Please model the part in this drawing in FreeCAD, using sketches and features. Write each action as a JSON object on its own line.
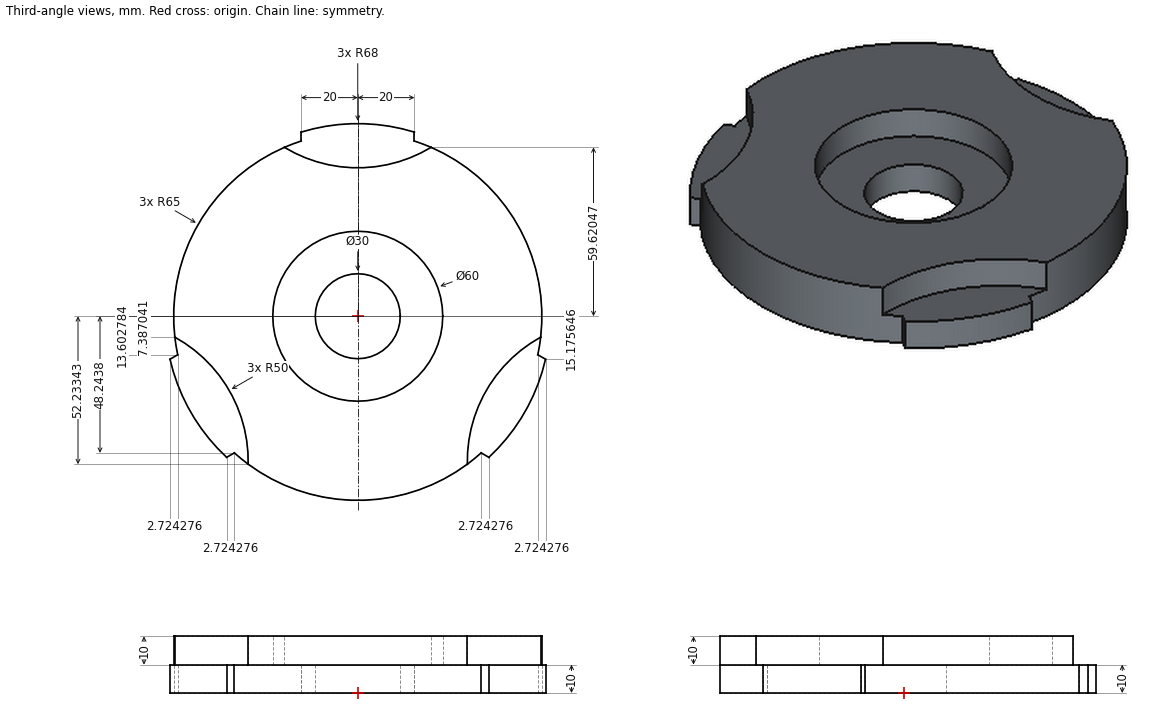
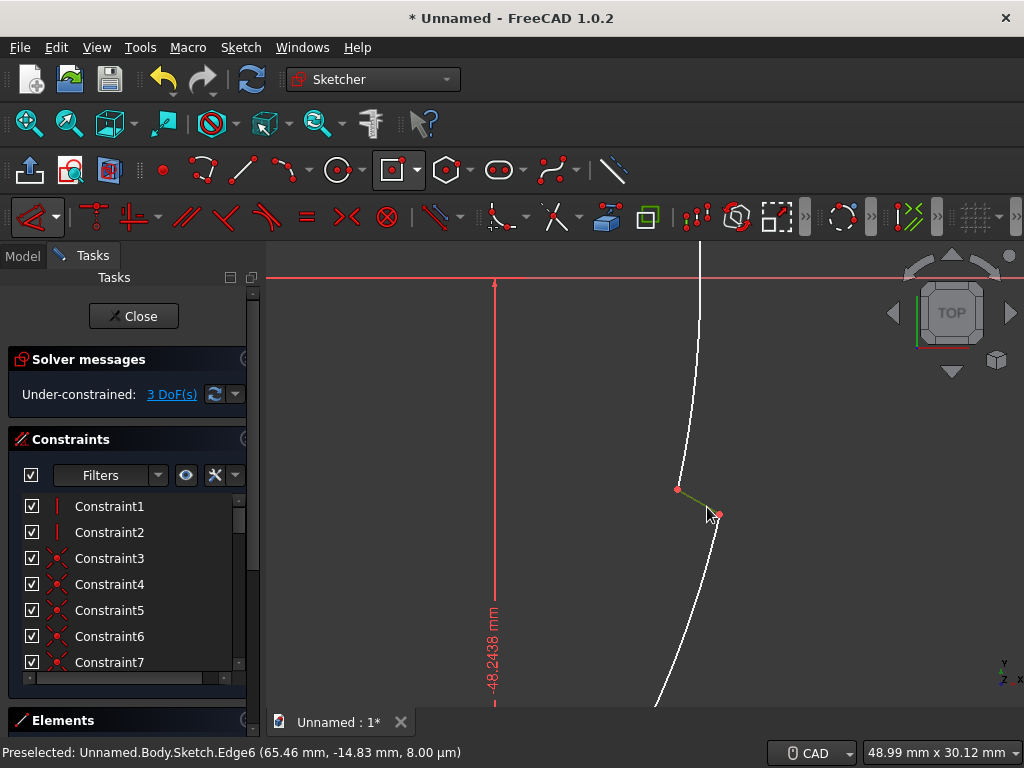
{"action": "key", "text": "l"}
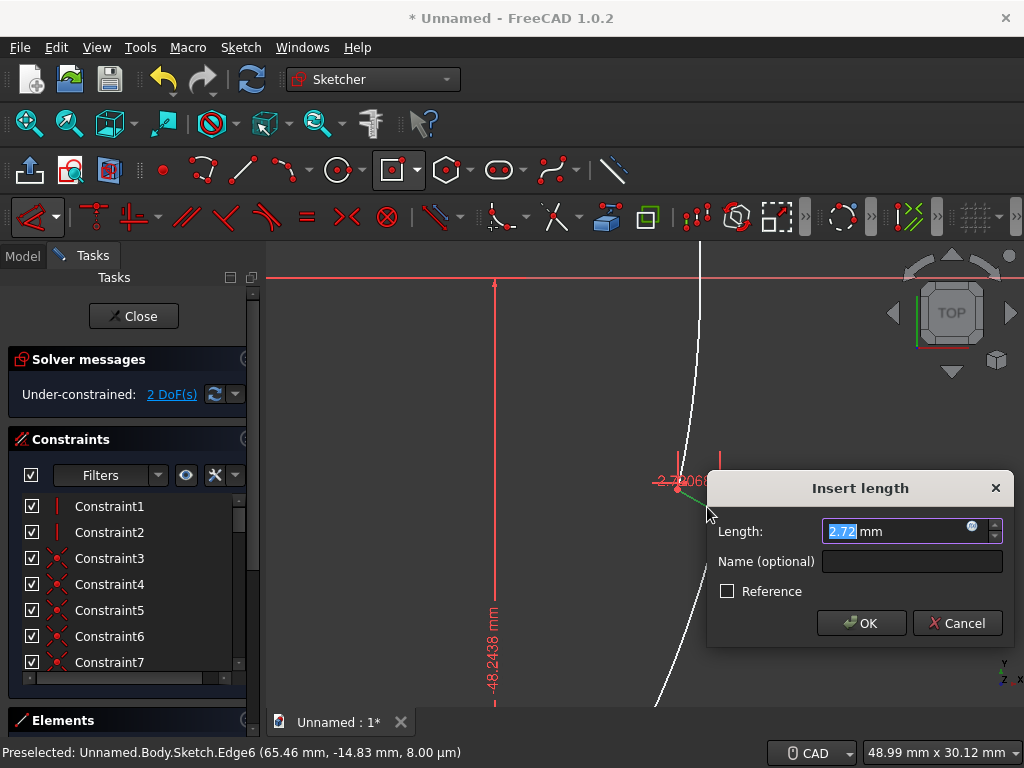
{"action": "type", "text": "2.724276"}
{"action": "key", "text": "Return"}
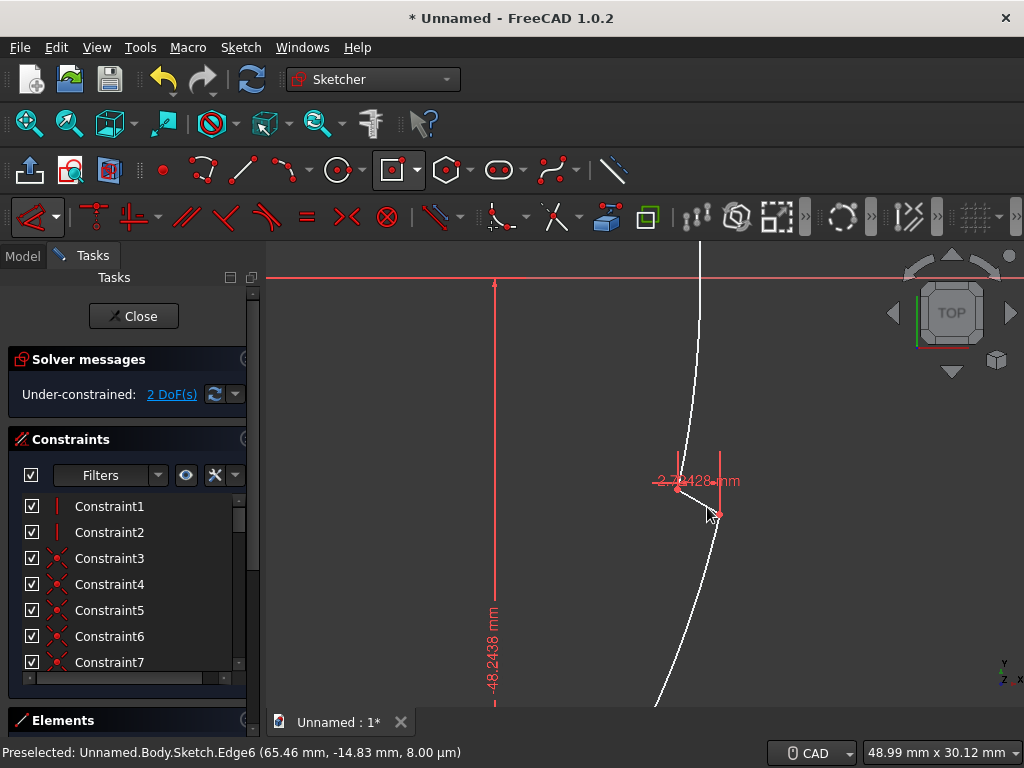
{"action": "scroll", "coordinate": [715, 508], "scroll_direction": "down", "scroll_amount": 10}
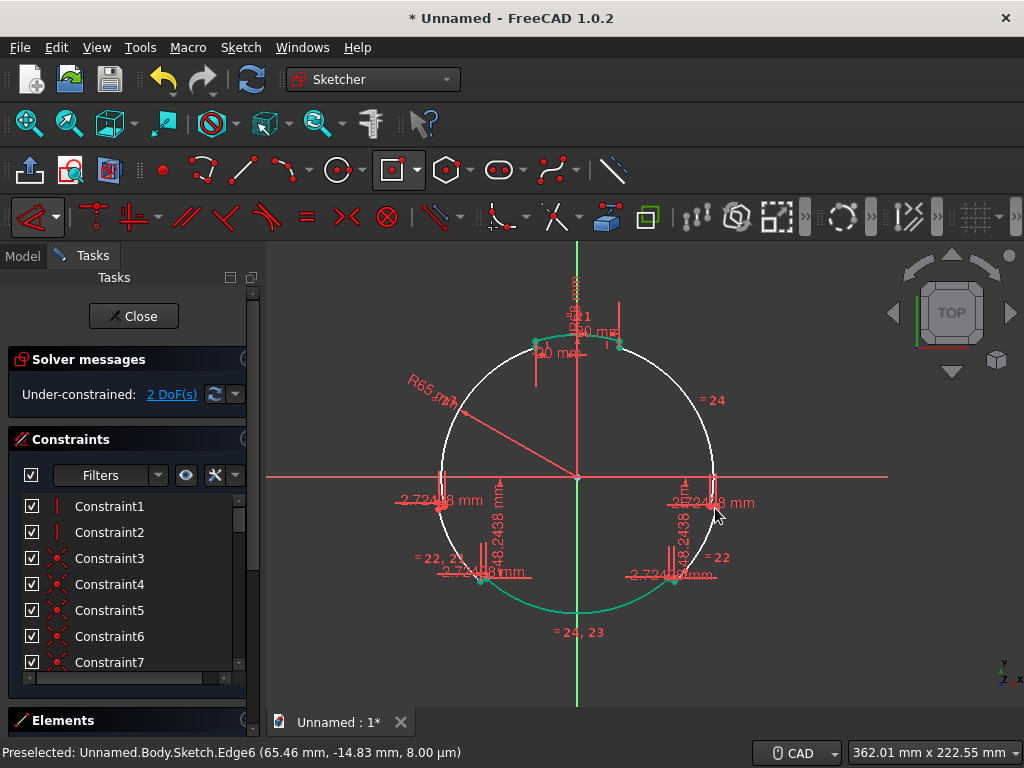
{"action": "scroll", "coordinate": [445, 507], "scroll_direction": "up", "scroll_amount": 4}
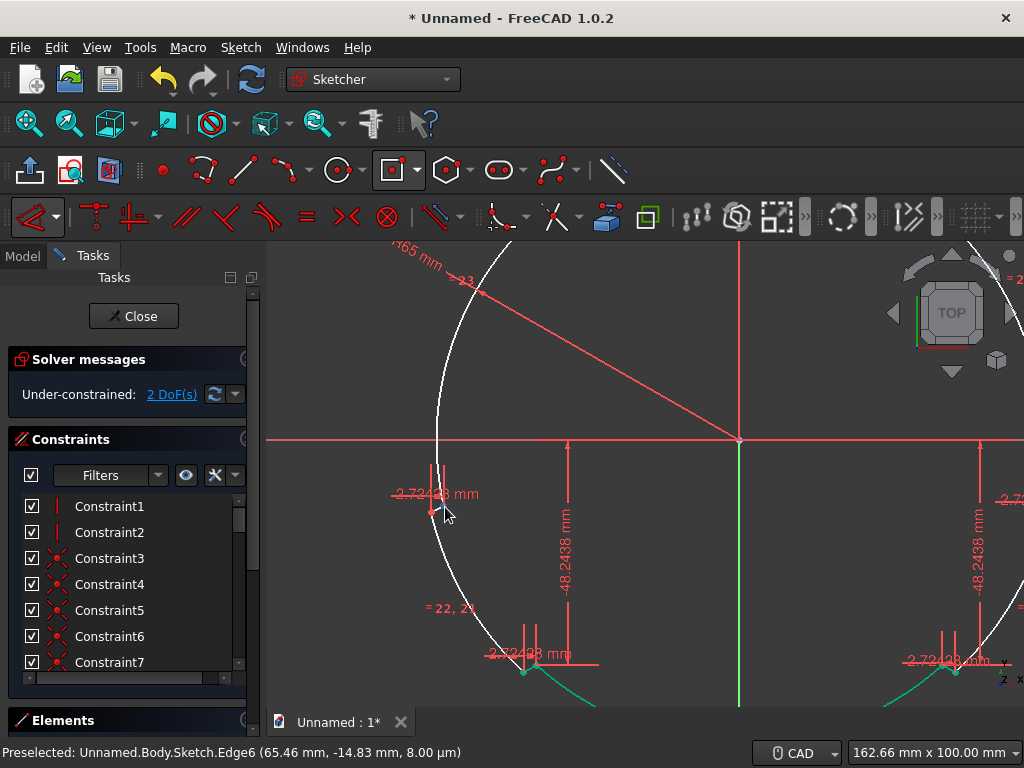
{"action": "left_click", "coordinate": [444, 506]}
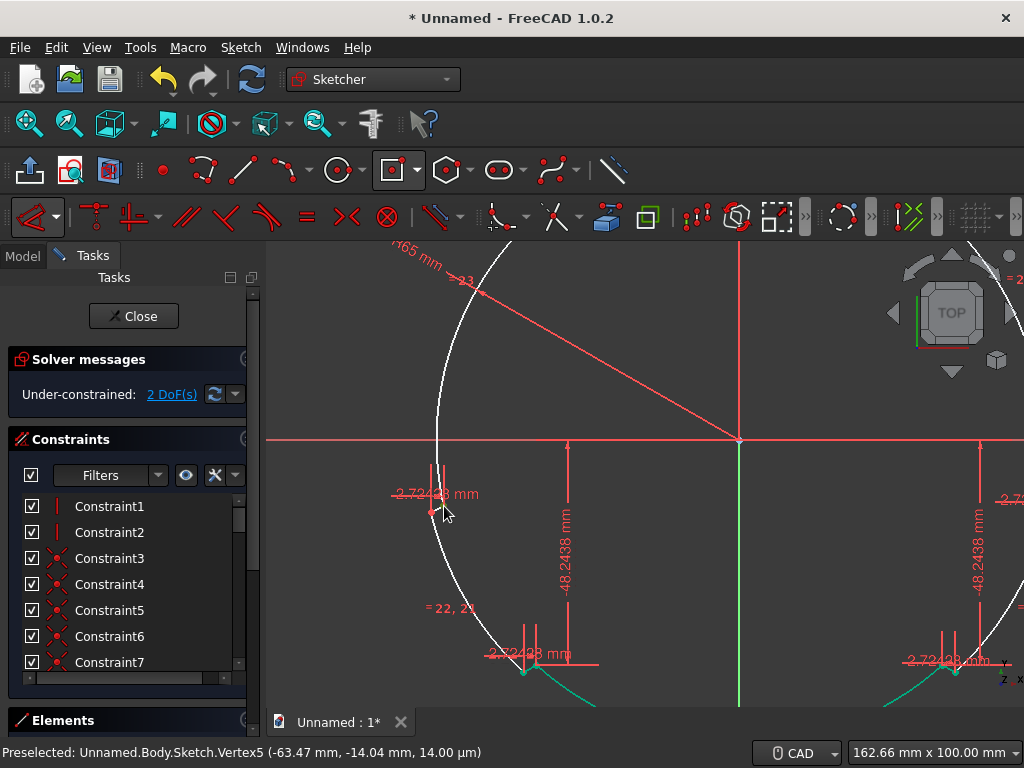
{"action": "key", "text": "i"}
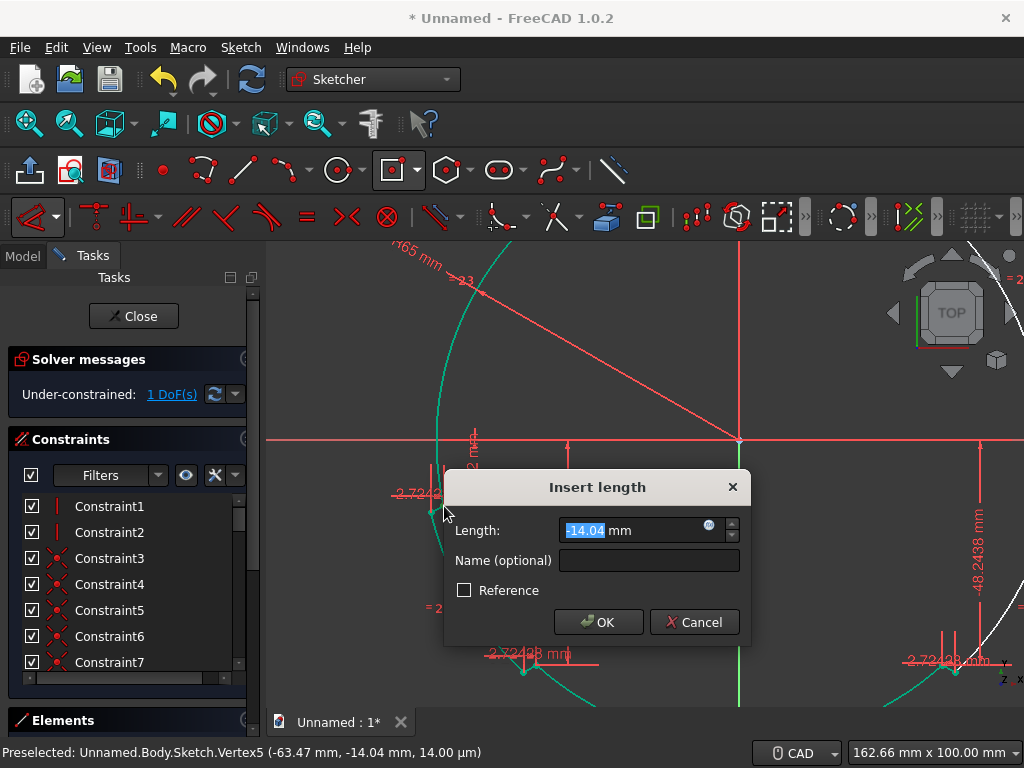
{"action": "type", "text": "-13.602784"}
{"action": "key", "text": "Return"}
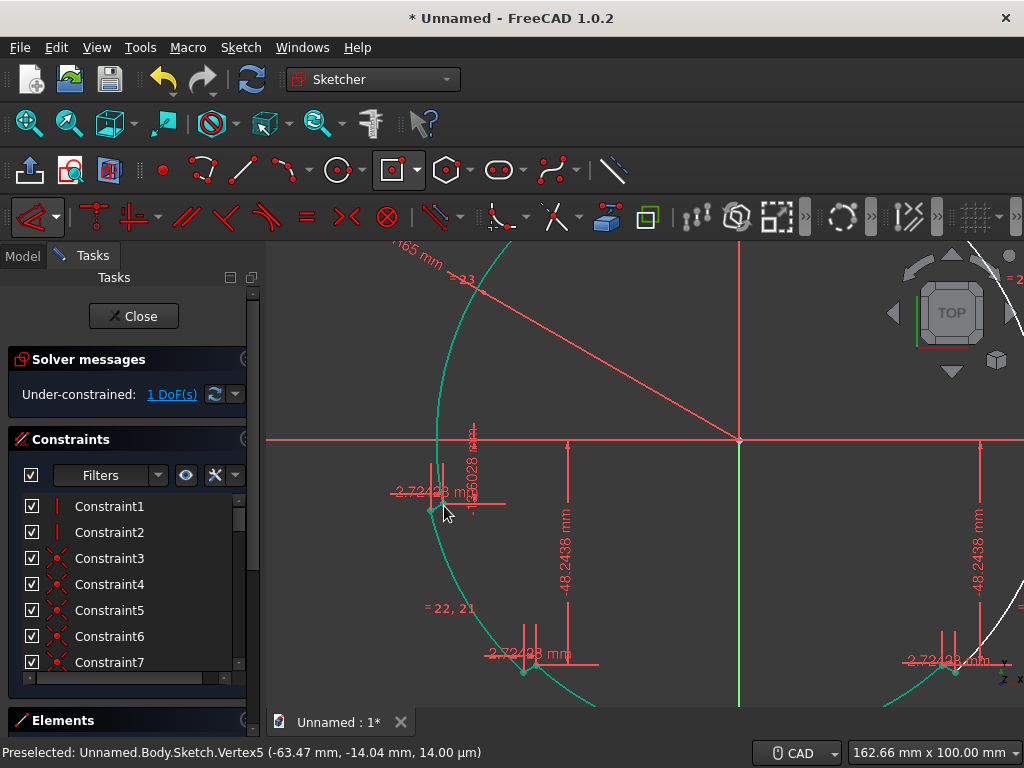
{"action": "scroll", "coordinate": [444, 507], "scroll_direction": "down", "scroll_amount": 4}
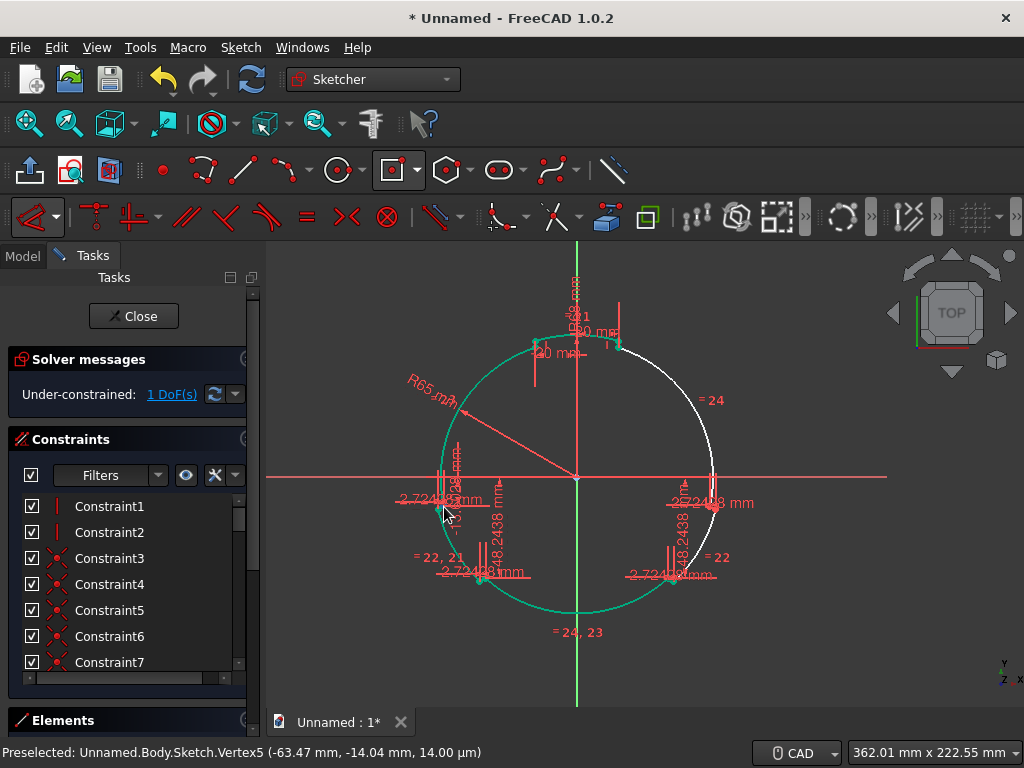
{"action": "scroll", "coordinate": [716, 509], "scroll_direction": "up", "scroll_amount": 4}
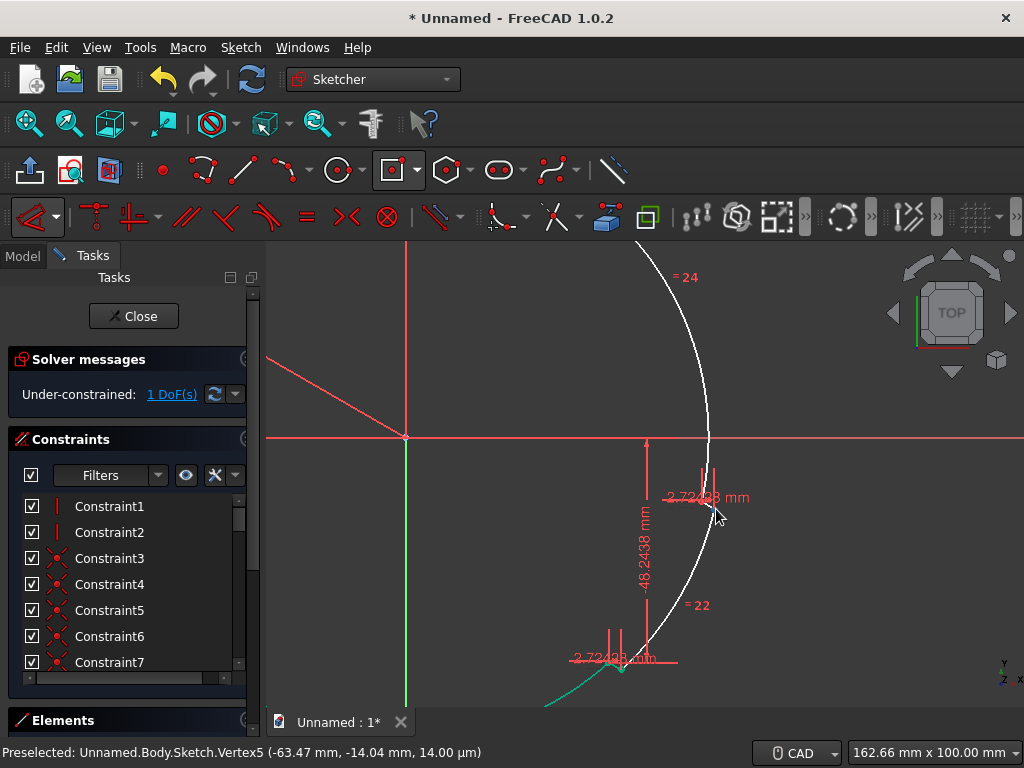
{"action": "left_click", "coordinate": [714, 509]}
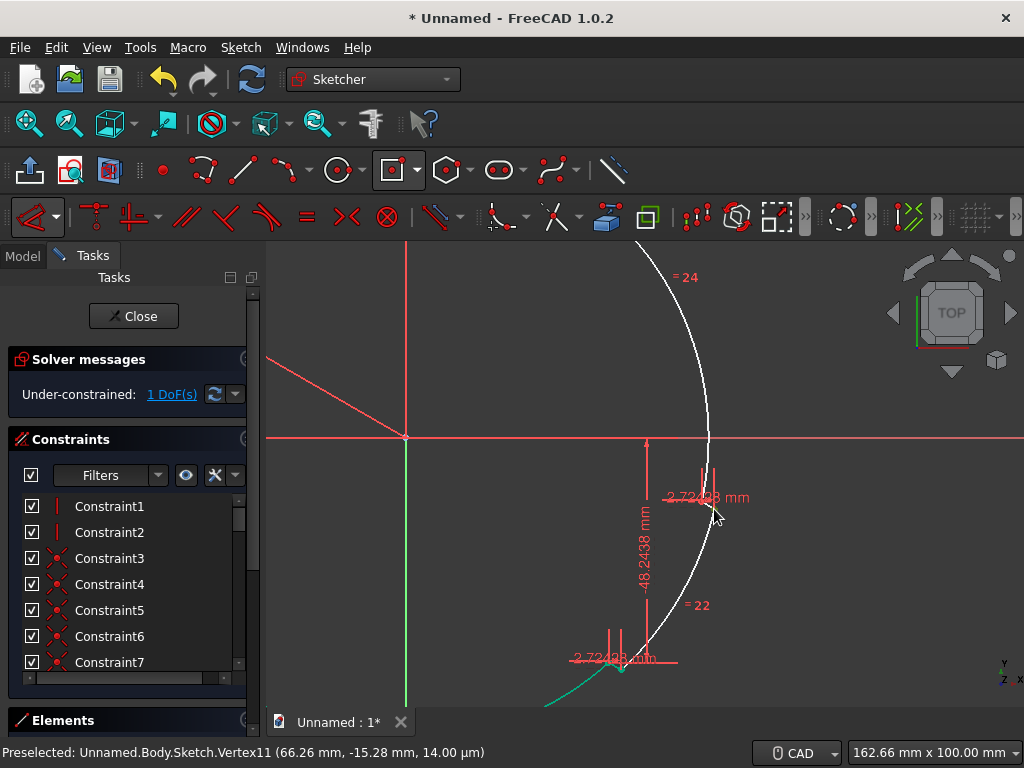
{"action": "left_click", "coordinate": [58, 218]}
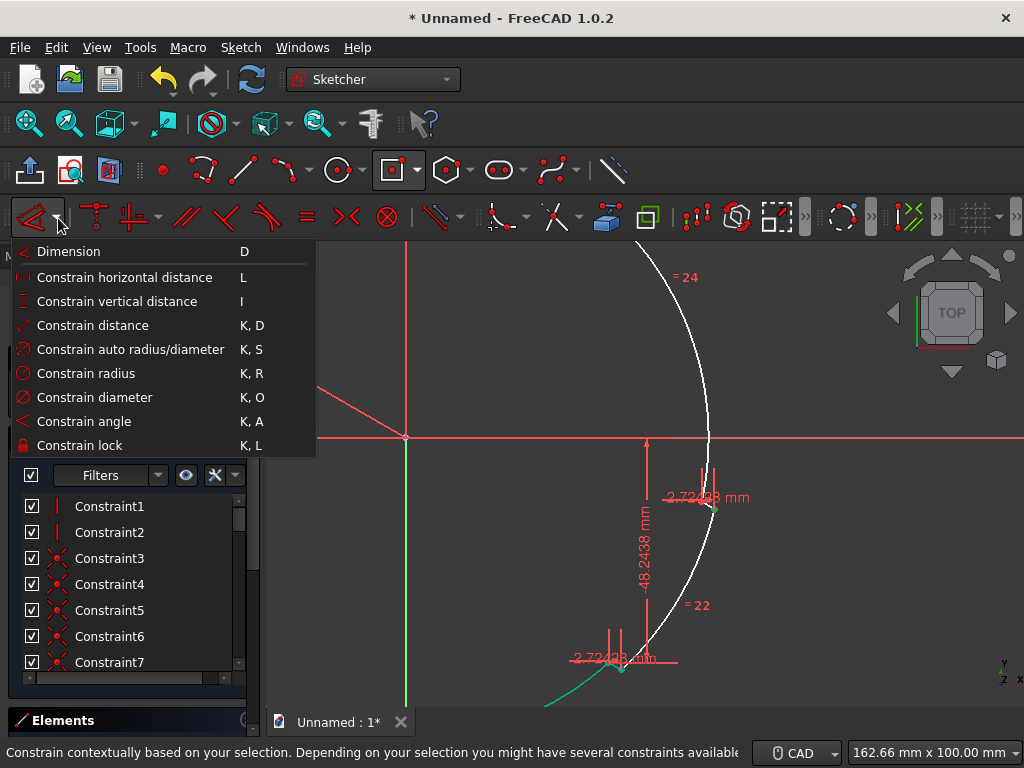
{"action": "left_click", "coordinate": [164, 301]}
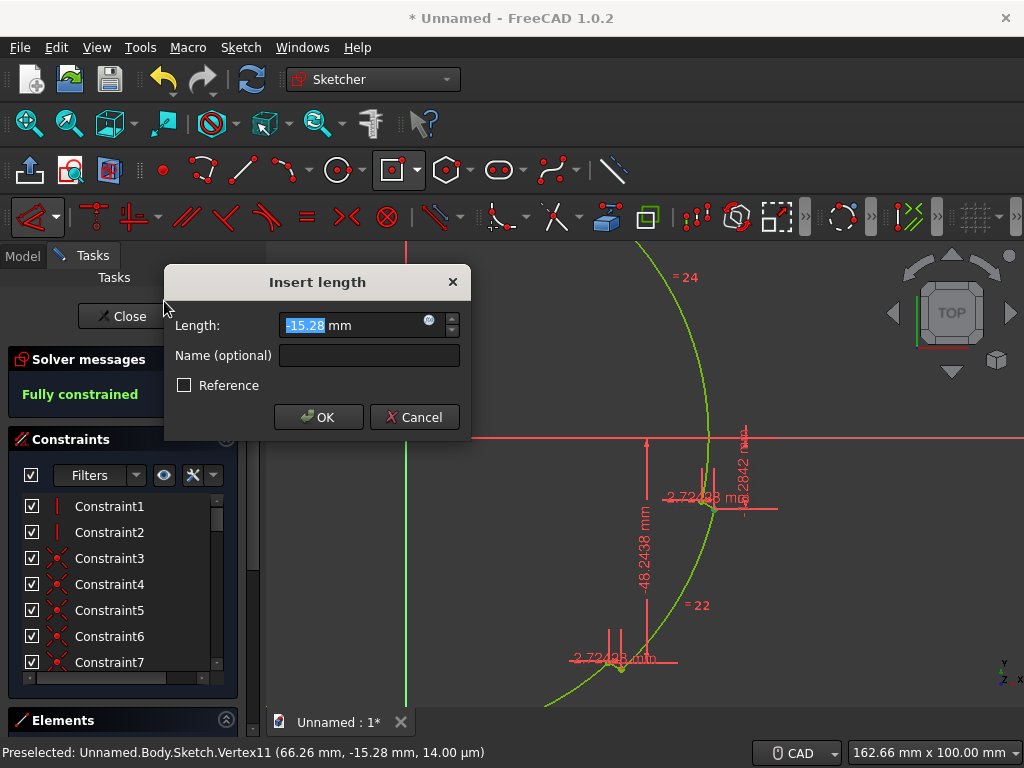
{"action": "type", "text": "-15.175646"}
{"action": "key", "text": "Return"}